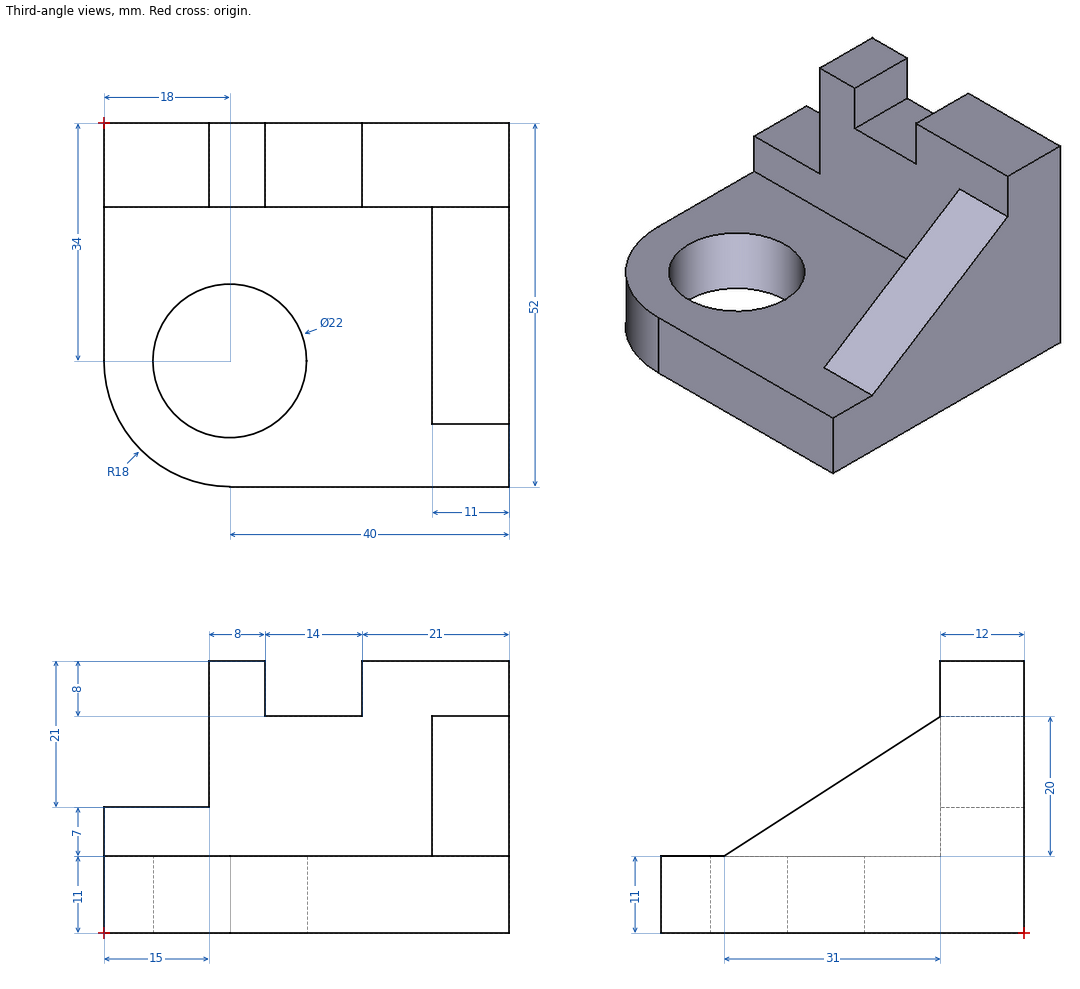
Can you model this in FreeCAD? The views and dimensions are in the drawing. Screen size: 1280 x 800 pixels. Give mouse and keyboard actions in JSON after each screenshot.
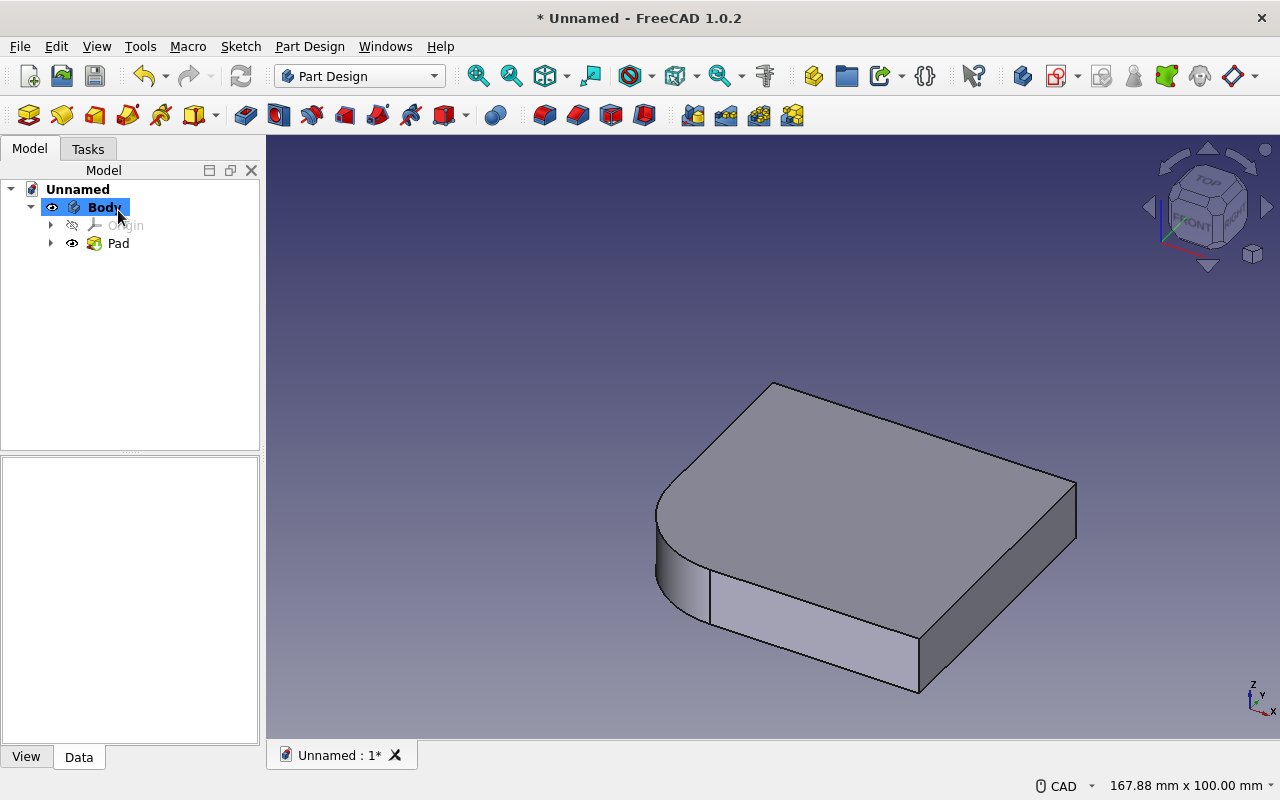
{"action": "key", "text": "4"}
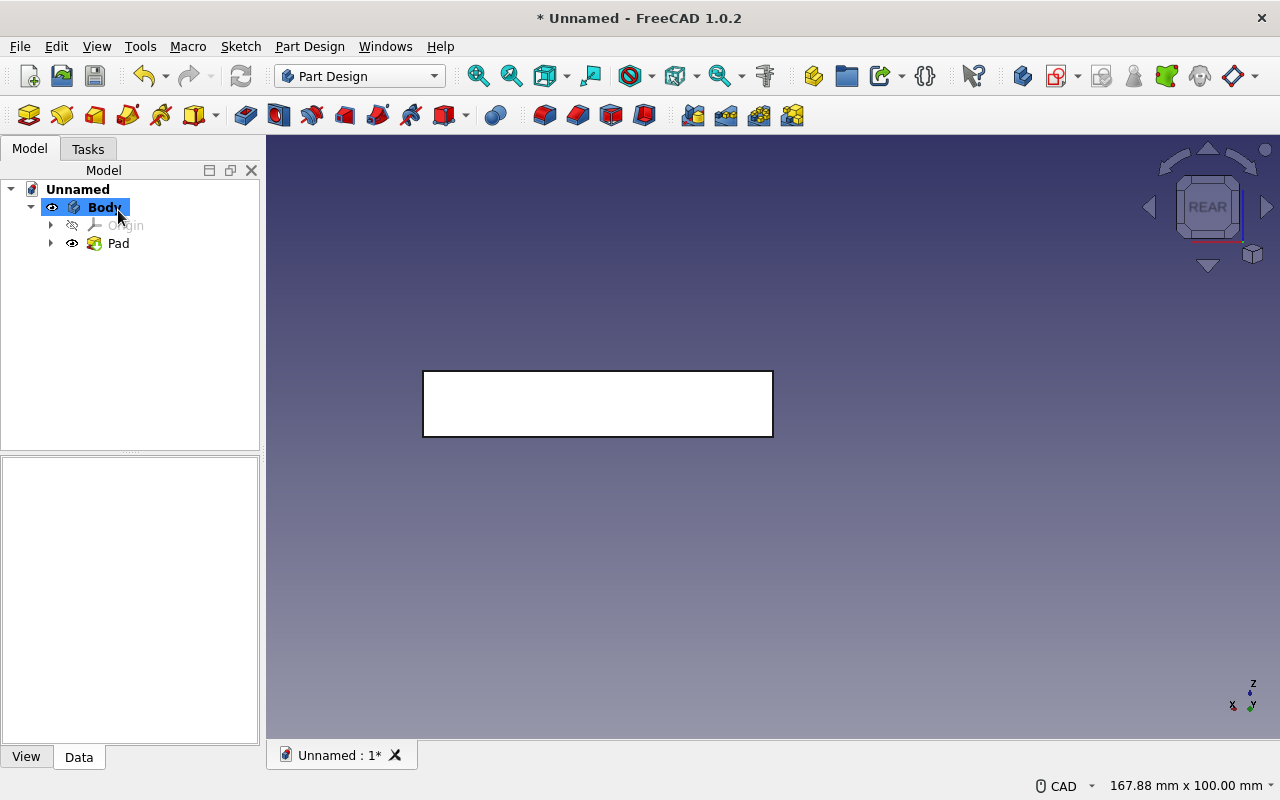
{"action": "left_click", "coordinate": [479, 76]}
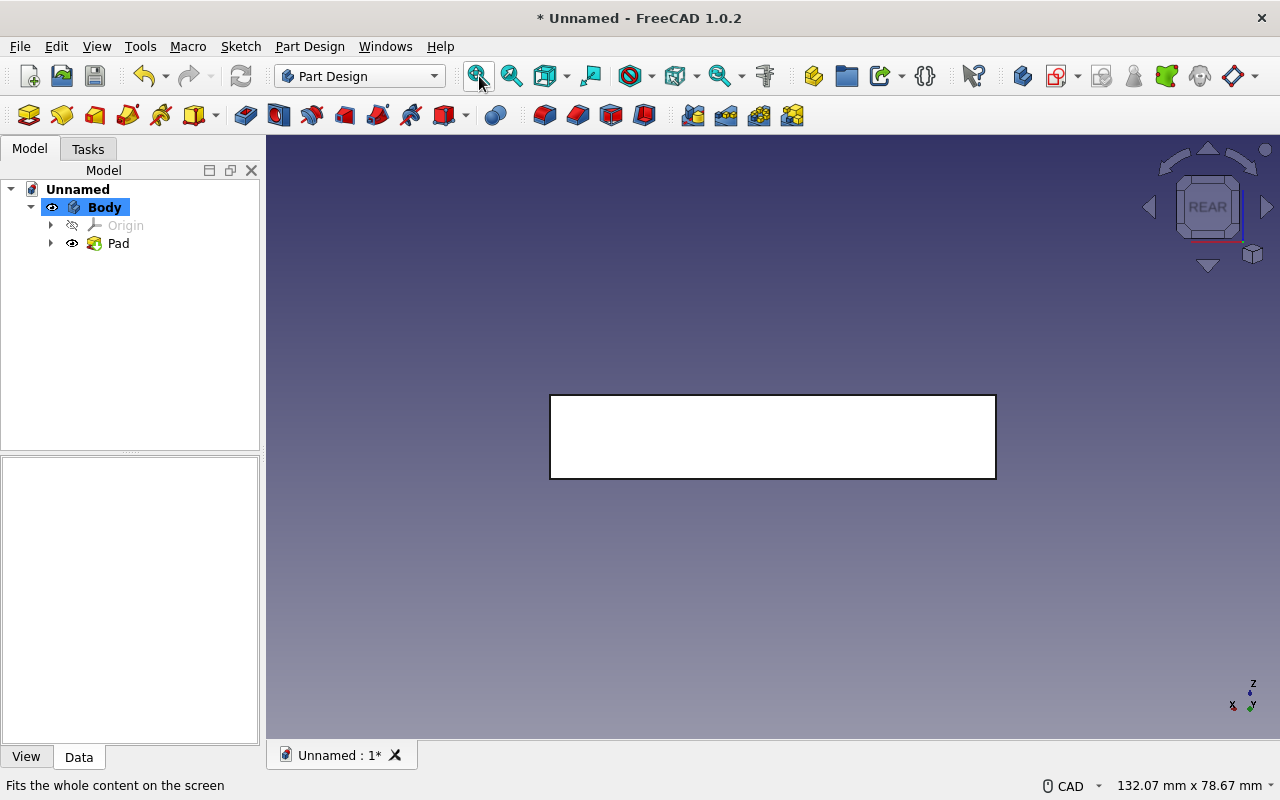
{"action": "left_click", "coordinate": [646, 436]}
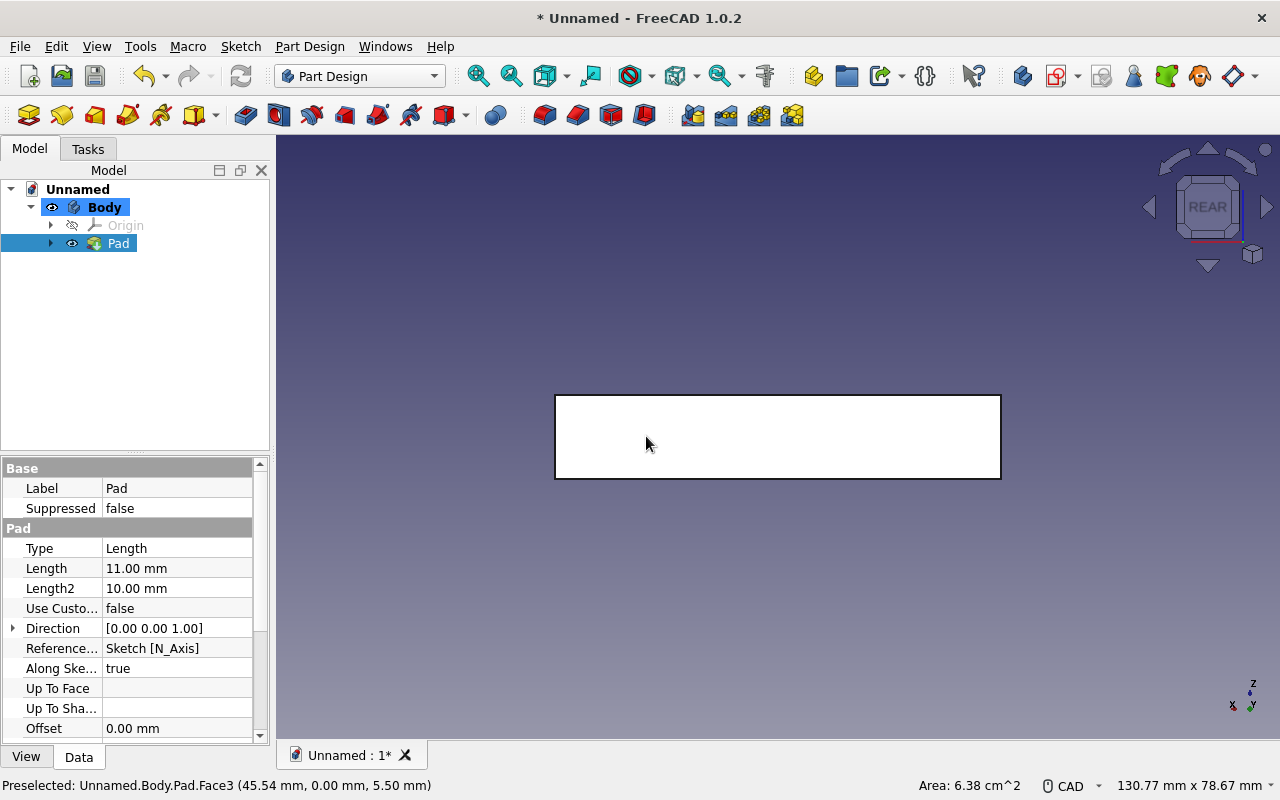
{"action": "left_click", "coordinate": [1056, 76]}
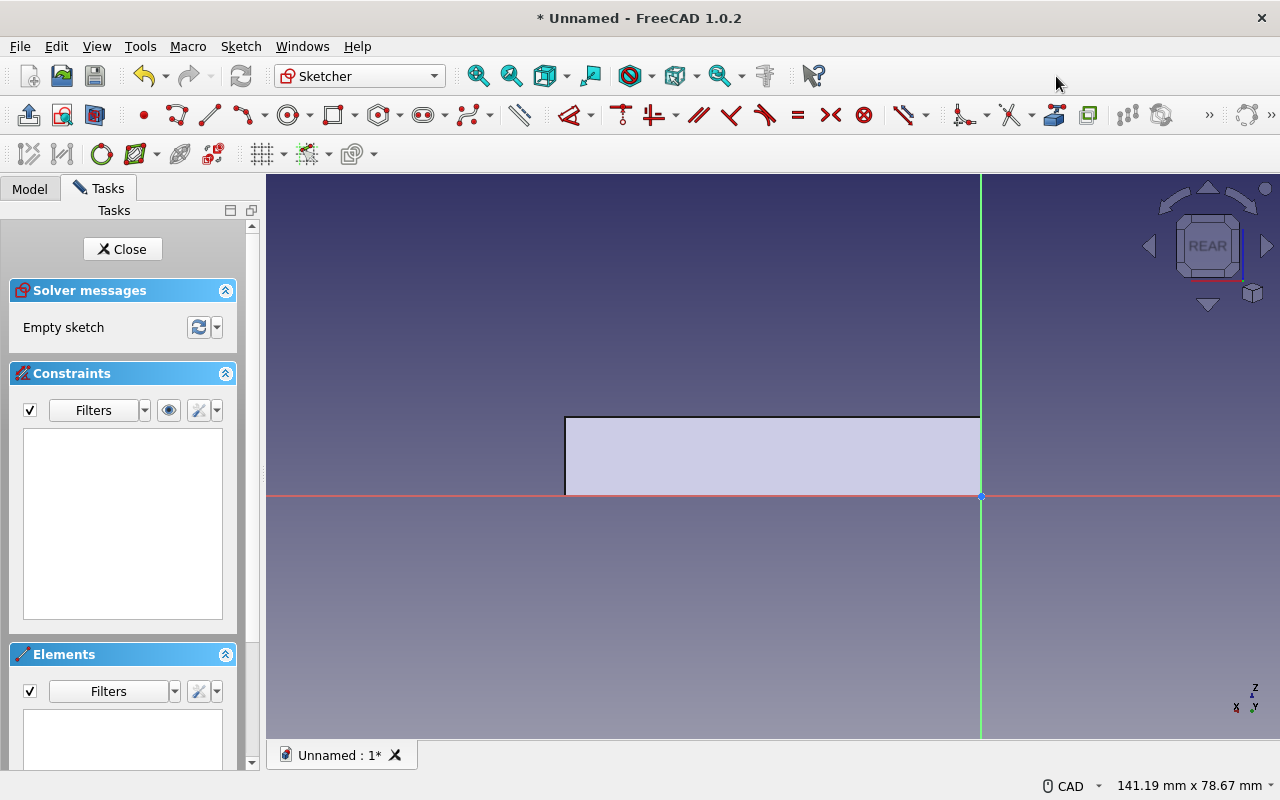
{"action": "scroll", "coordinate": [395, 711], "scroll_direction": "down", "scroll_amount": 1}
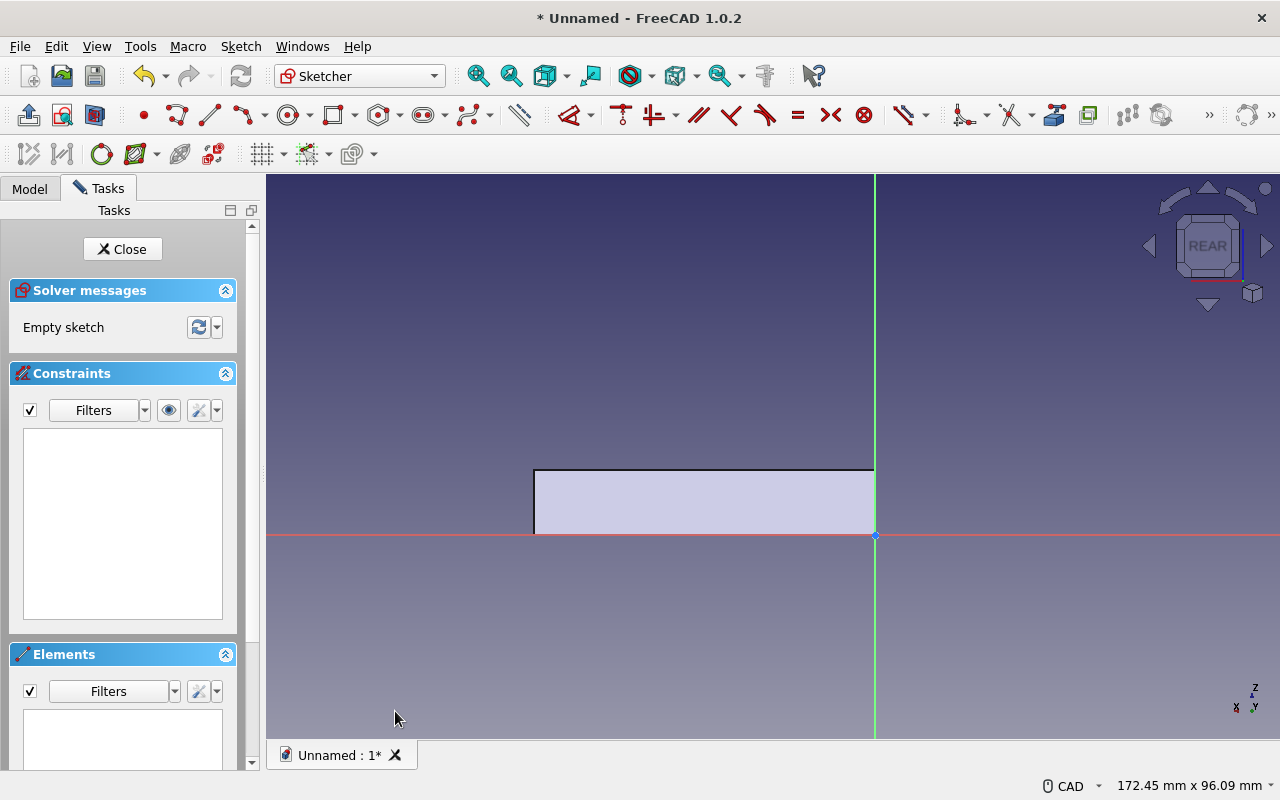
{"action": "scroll", "coordinate": [705, 347], "scroll_direction": "up", "scroll_amount": 2}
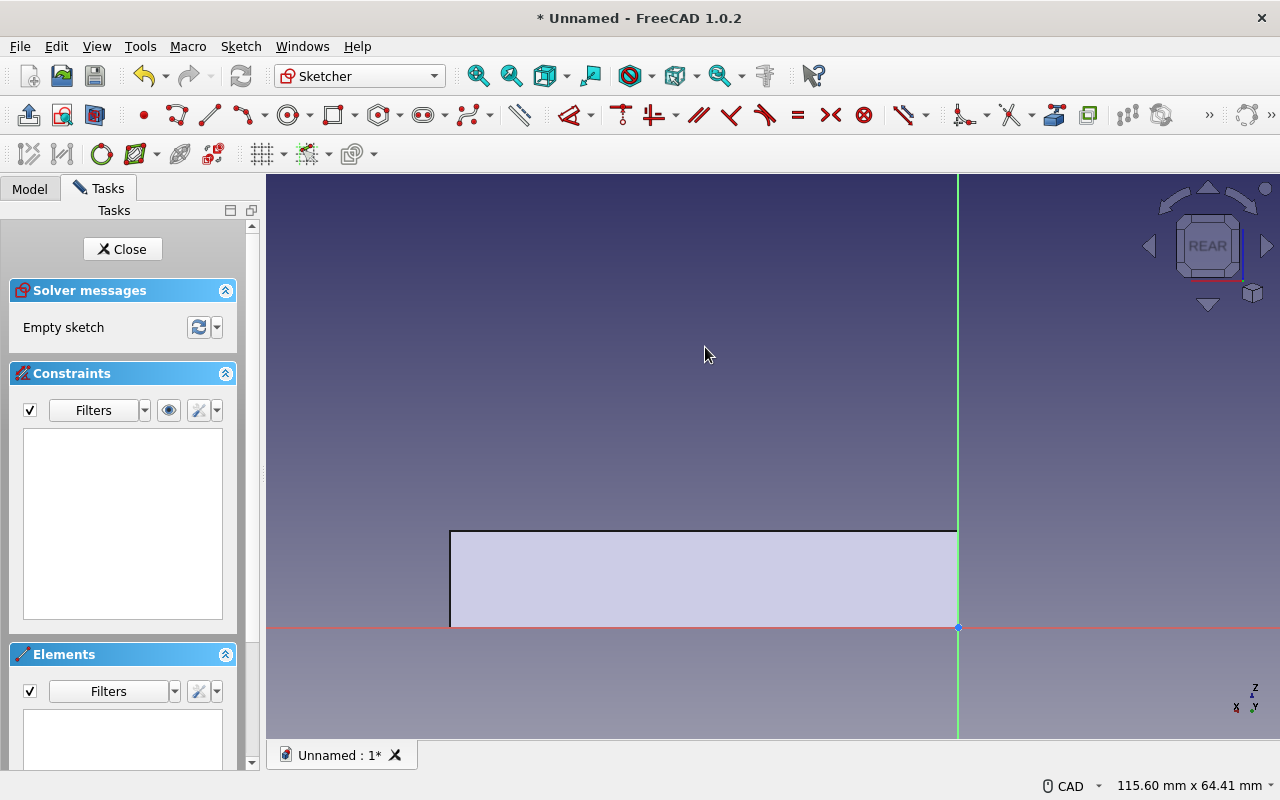
{"action": "left_click", "coordinate": [177, 116]}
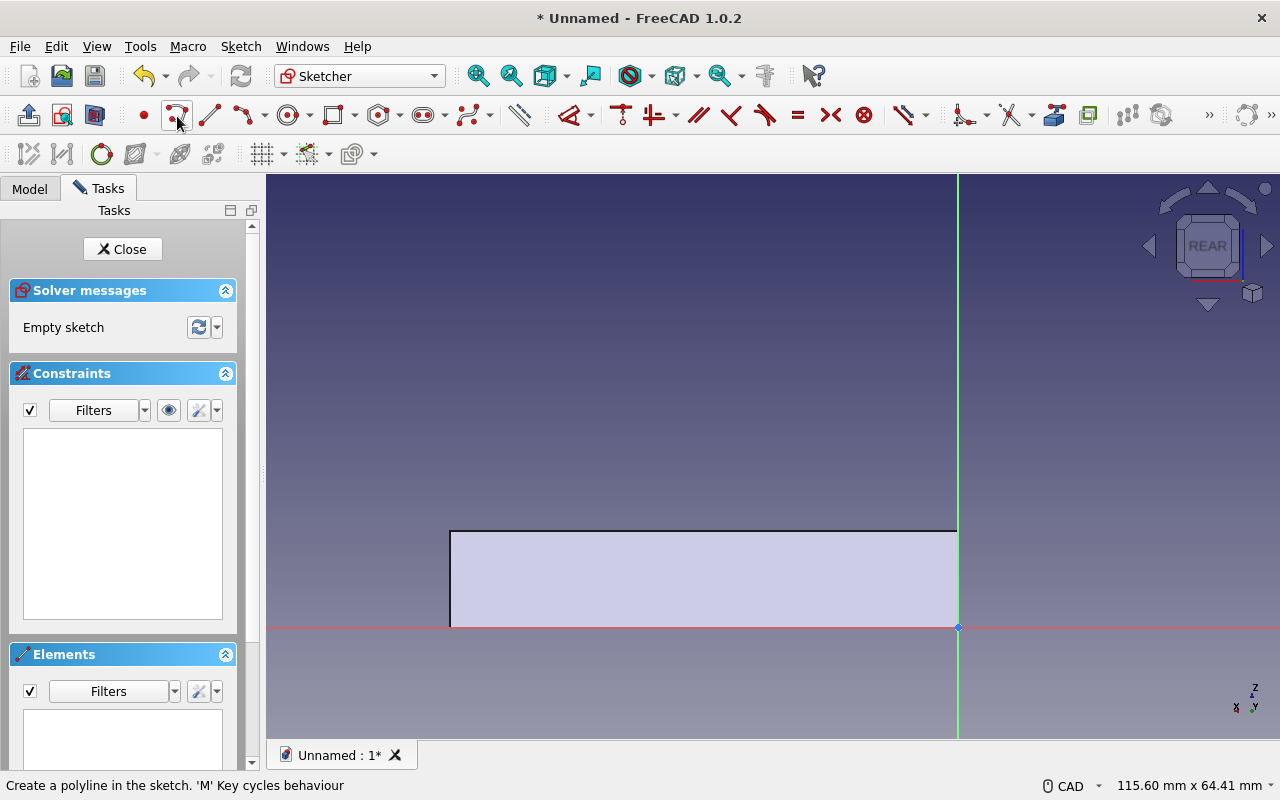
{"action": "left_click", "coordinate": [958, 531]}
{"action": "left_click", "coordinate": [949, 470]}
{"action": "left_click", "coordinate": [827, 470]}
{"action": "left_click", "coordinate": [827, 285]}
{"action": "left_click", "coordinate": [757, 285]}
{"action": "left_click", "coordinate": [757, 356]}
{"action": "left_click", "coordinate": [634, 356]}
{"action": "left_click", "coordinate": [634, 285]}
{"action": "left_click", "coordinate": [450, 285]}
{"action": "left_click", "coordinate": [450, 531]}
{"action": "left_click", "coordinate": [958, 532]}
{"action": "key", "text": "Escape"}
{"action": "key", "text": "Escape"}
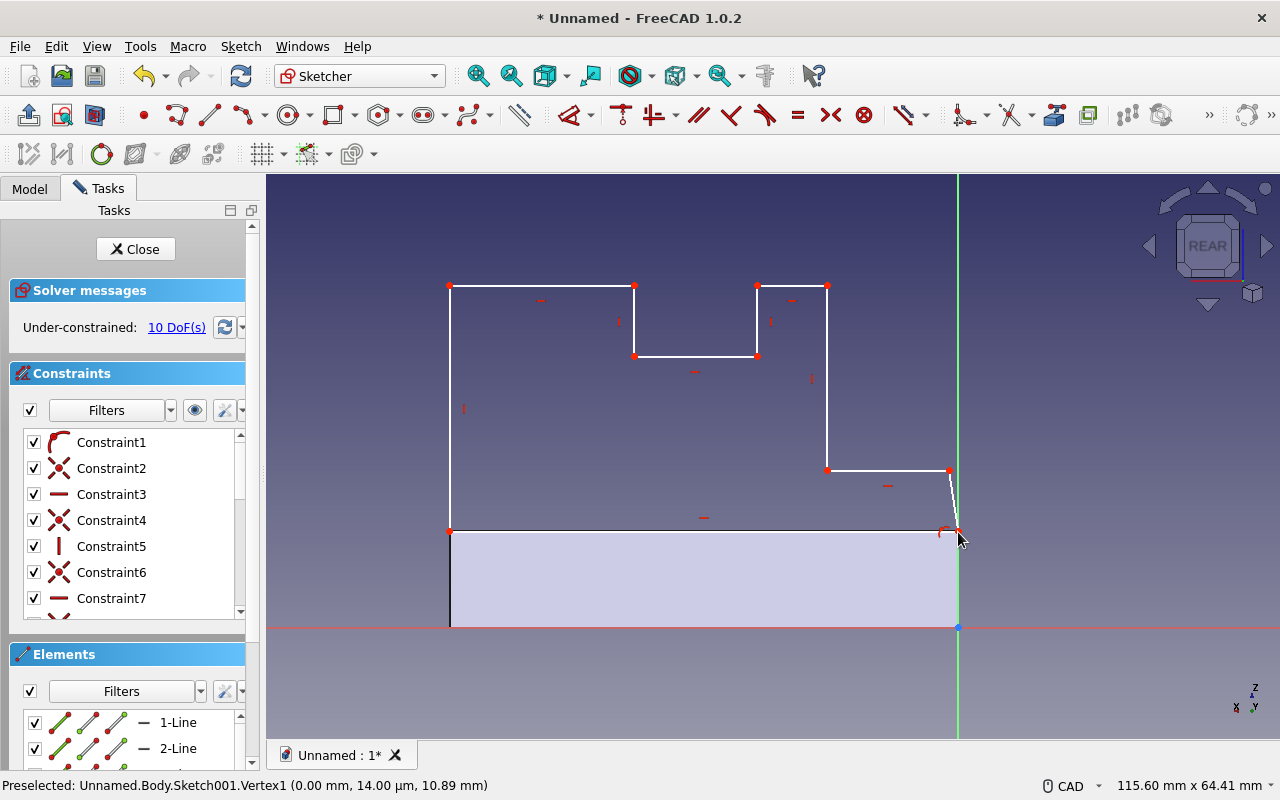
{"action": "left_click", "coordinate": [956, 514]}